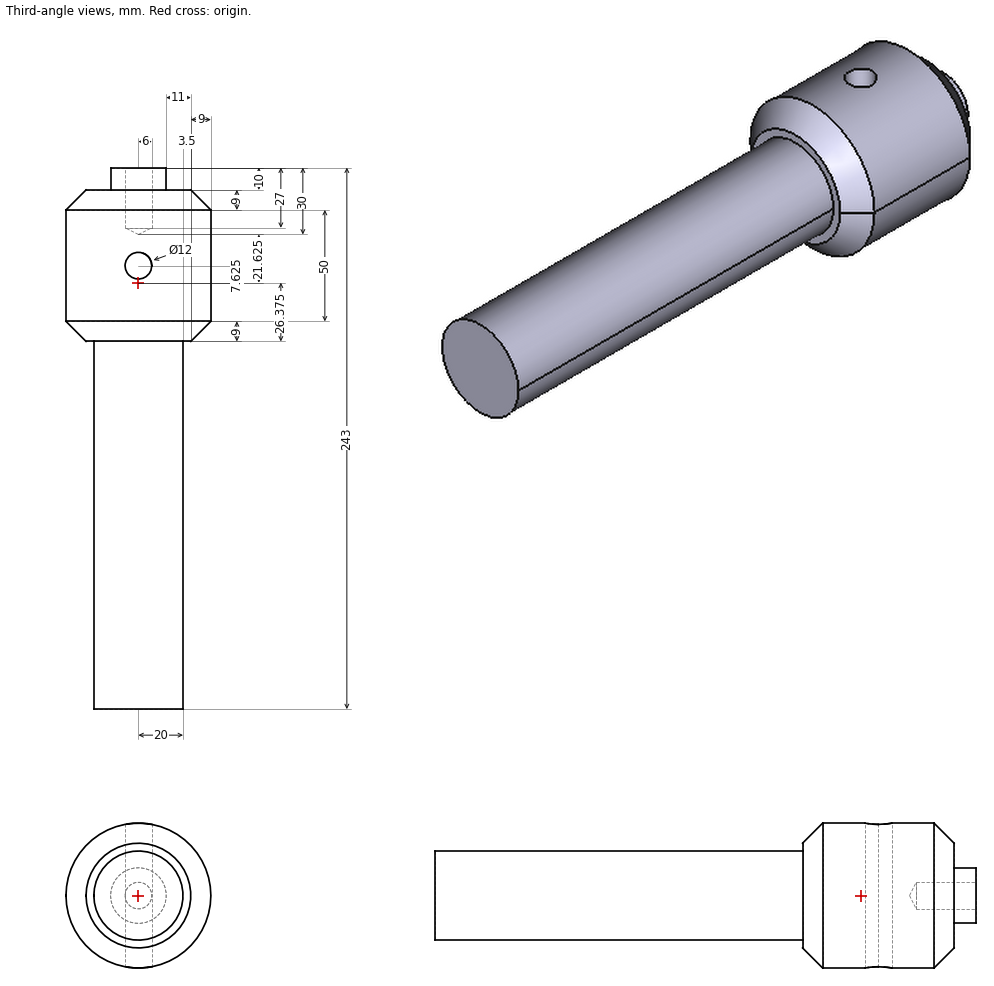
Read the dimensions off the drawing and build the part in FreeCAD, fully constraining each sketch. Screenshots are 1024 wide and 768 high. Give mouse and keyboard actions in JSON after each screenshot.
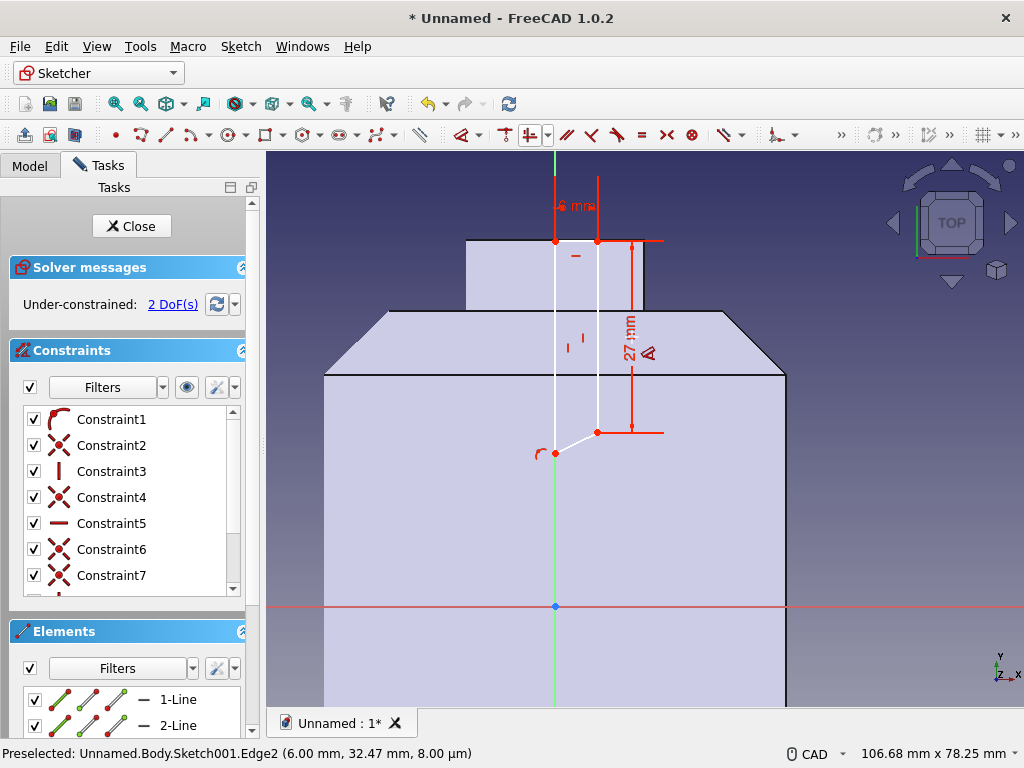
{"action": "left_click", "coordinate": [555, 305]}
{"action": "left_click", "coordinate": [521, 348]}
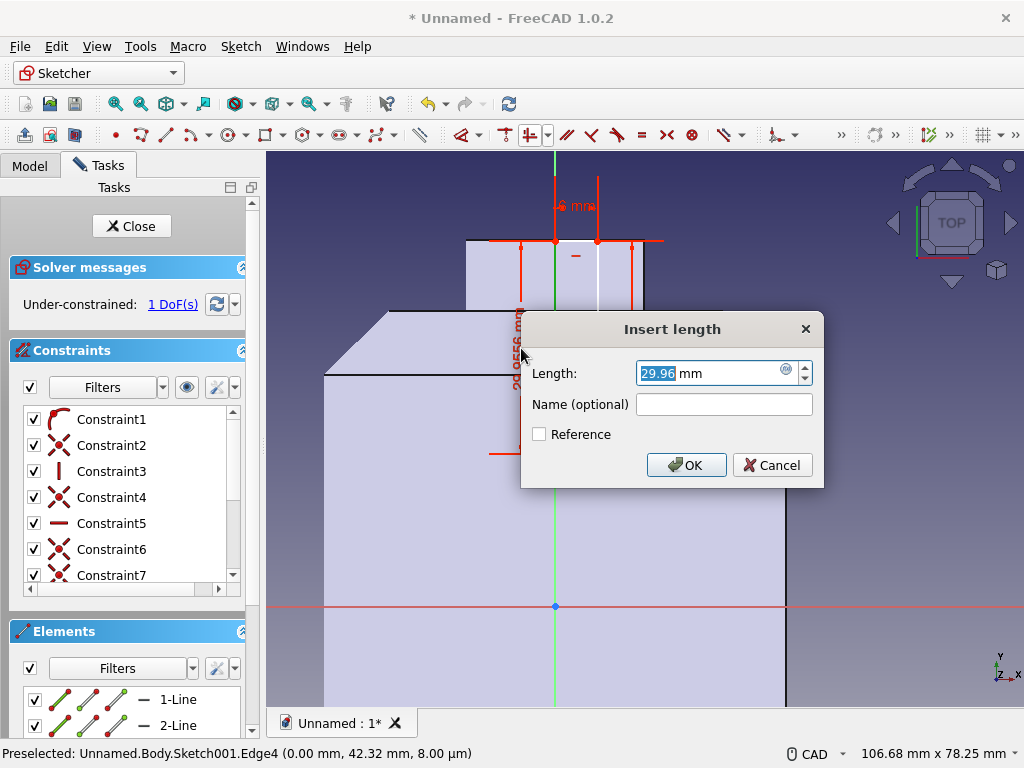
{"action": "type", "text": "30"}
{"action": "key", "text": "Return"}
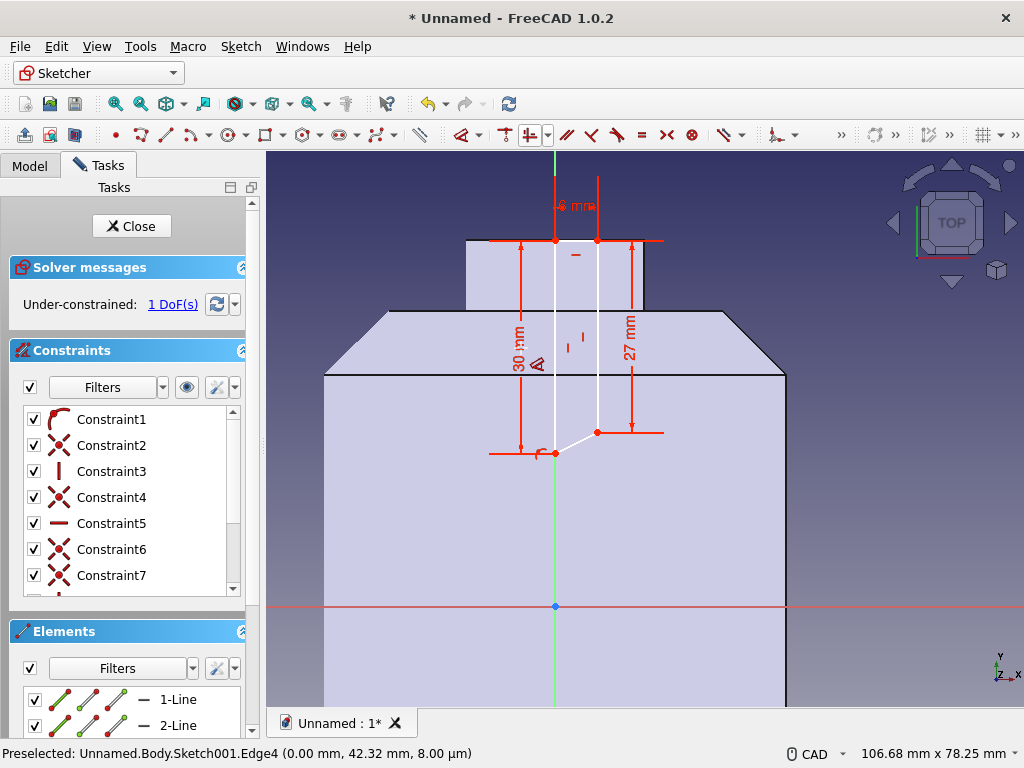
{"action": "left_click", "coordinate": [555, 454]}
{"action": "left_click", "coordinate": [521, 530]}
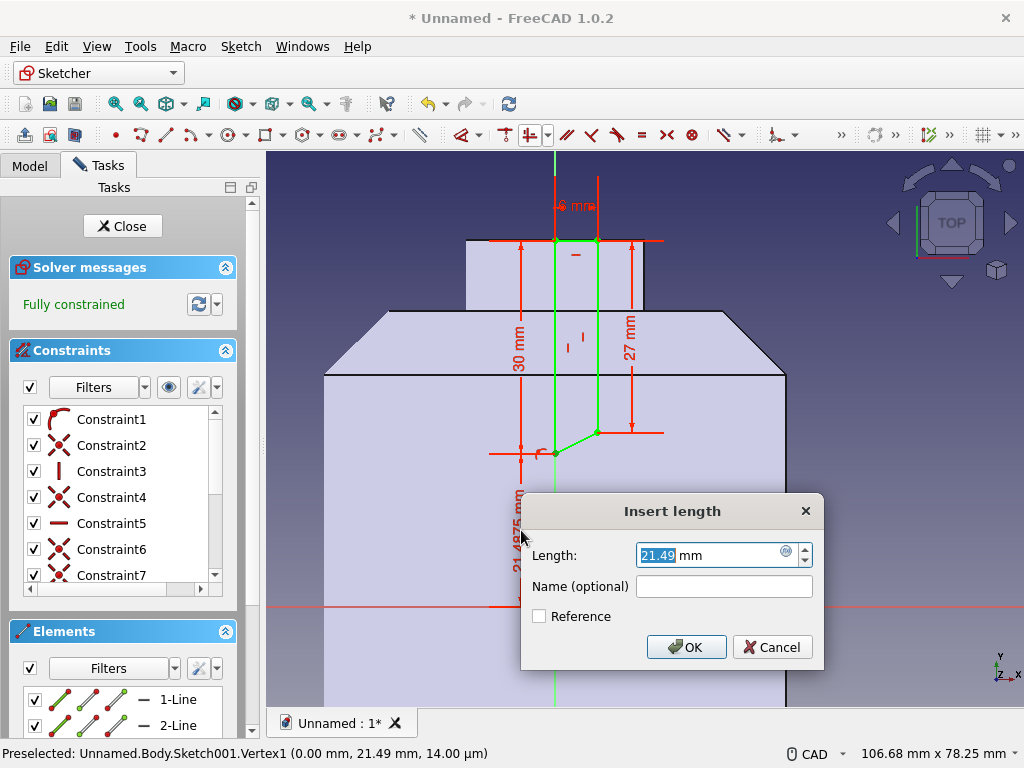
{"action": "type", "text": "21.625"}
{"action": "key", "text": "Return"}
{"action": "key", "text": "Escape"}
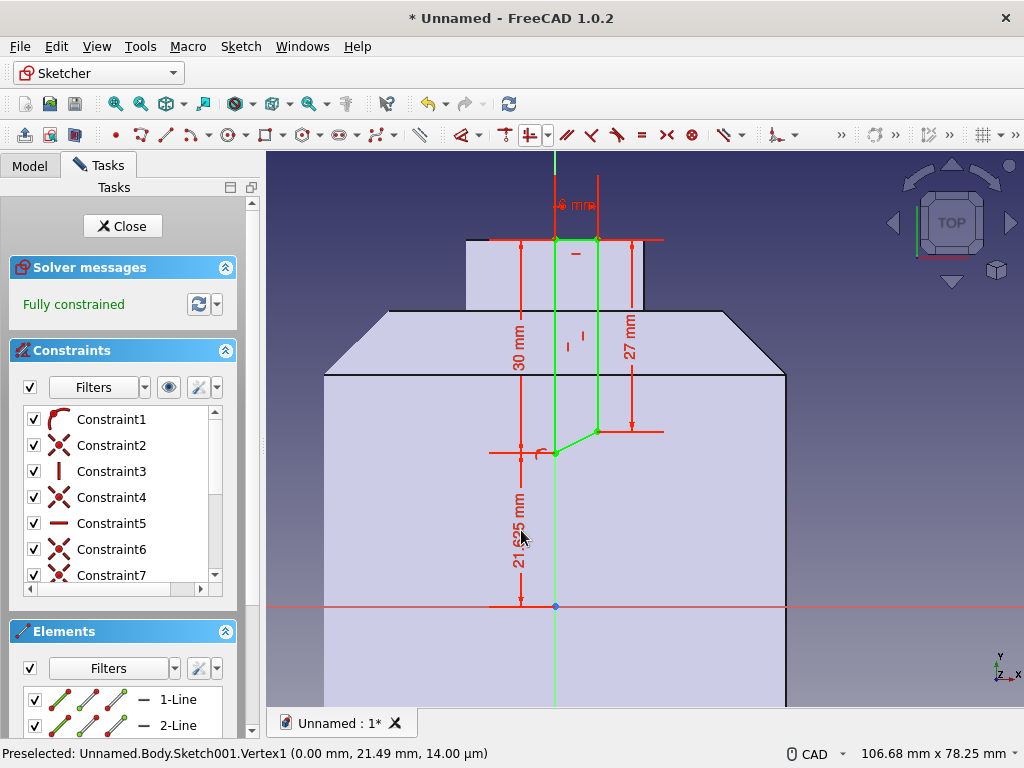
{"action": "left_click", "coordinate": [123, 226]}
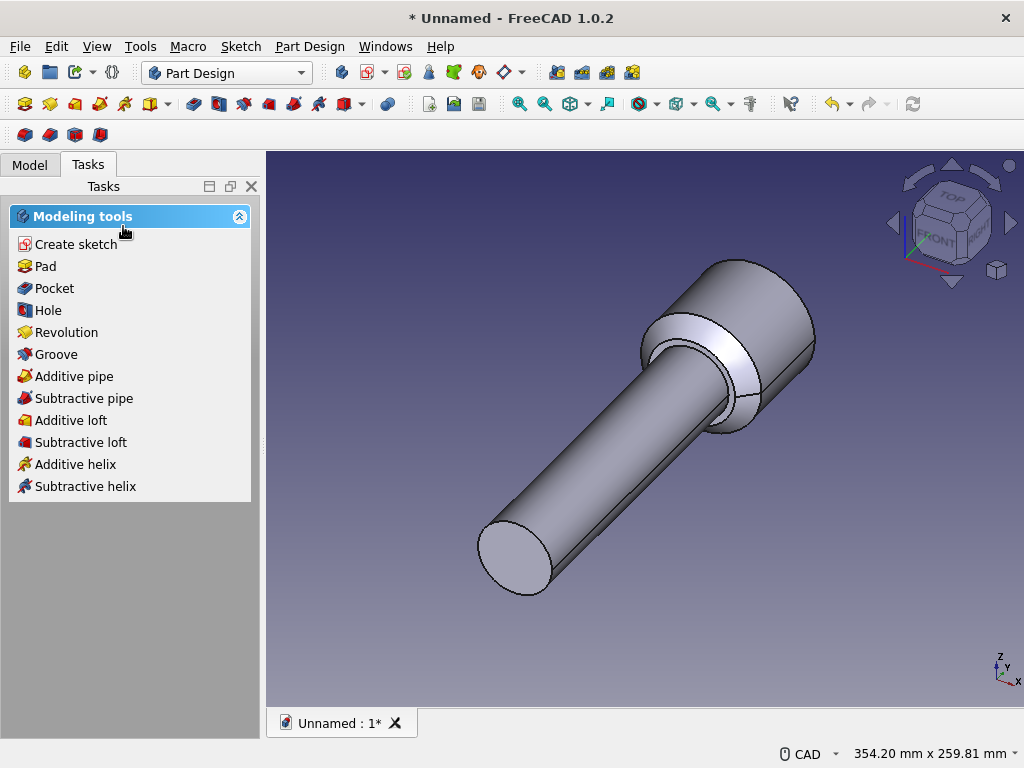
{"action": "left_click", "coordinate": [244, 104]}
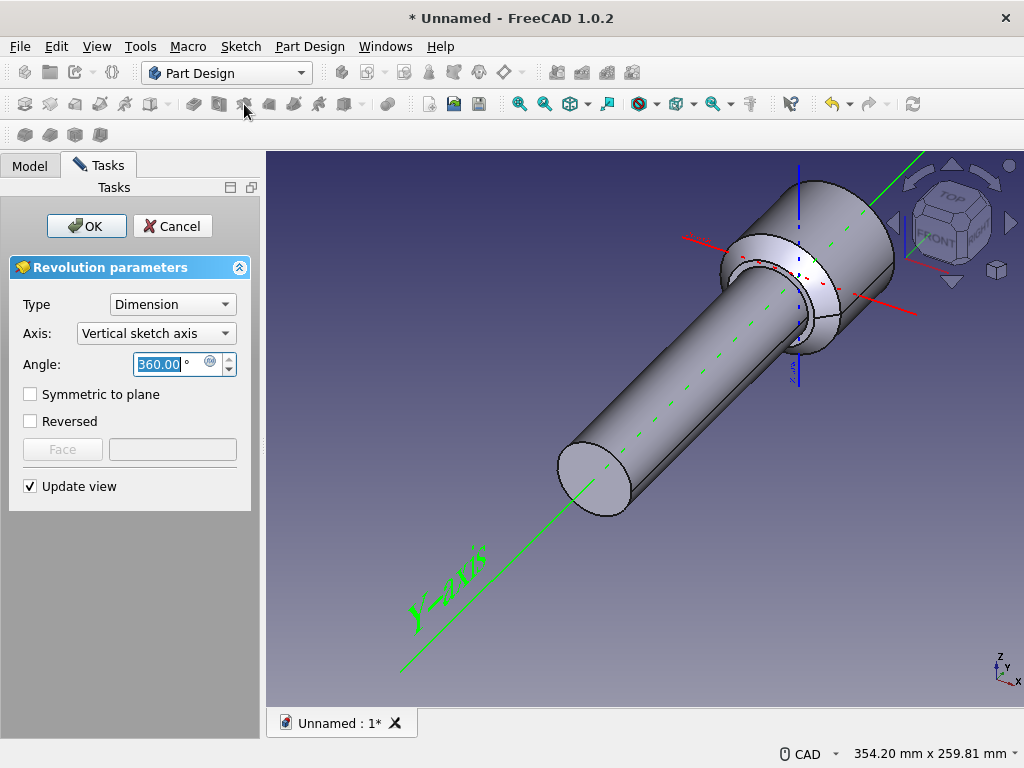
{"action": "left_click", "coordinate": [87, 226]}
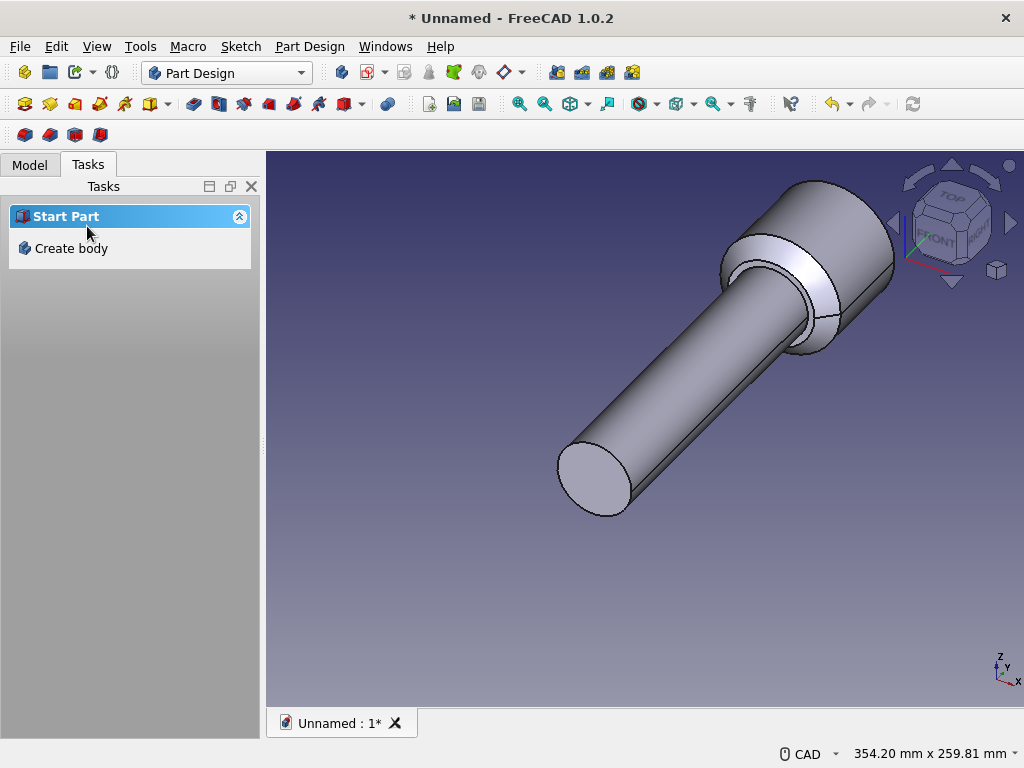
{"action": "left_click", "coordinate": [520, 104]}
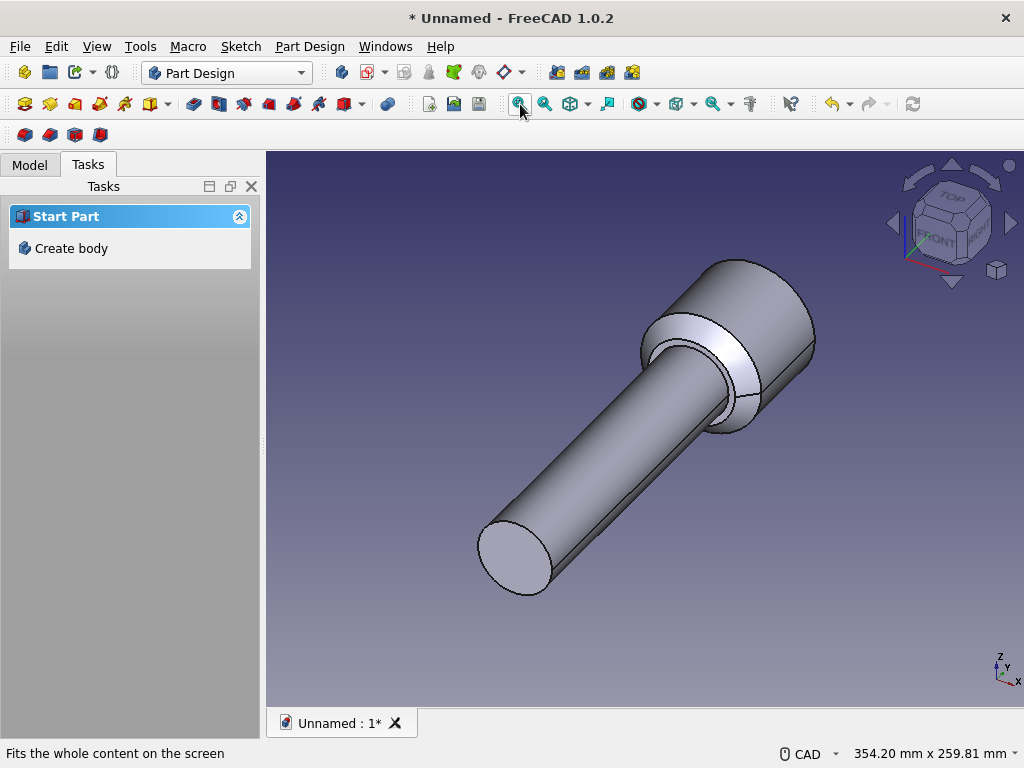
{"action": "left_click", "coordinate": [366, 72]}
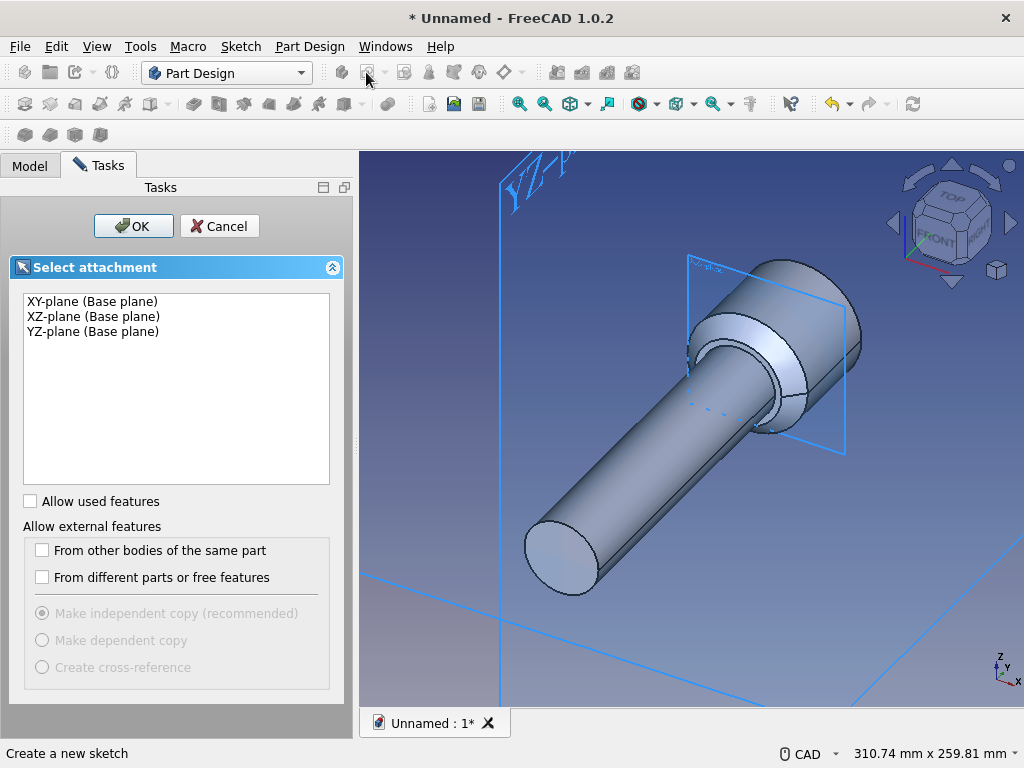
{"action": "left_click", "coordinate": [84, 302]}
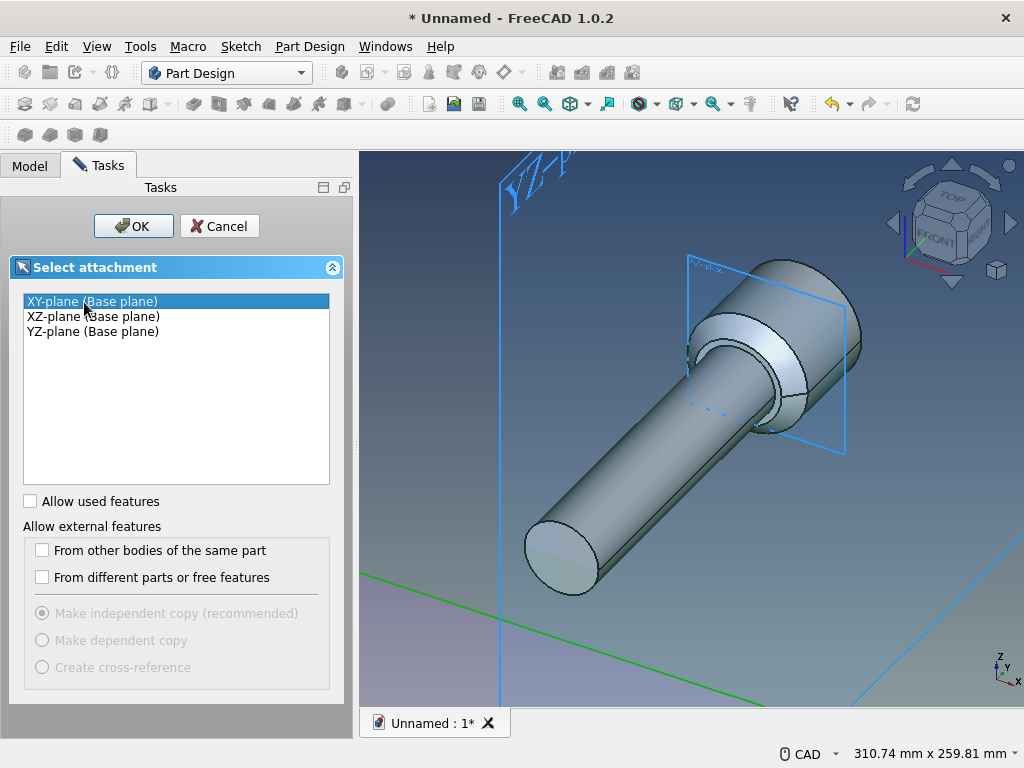
{"action": "left_click", "coordinate": [134, 226]}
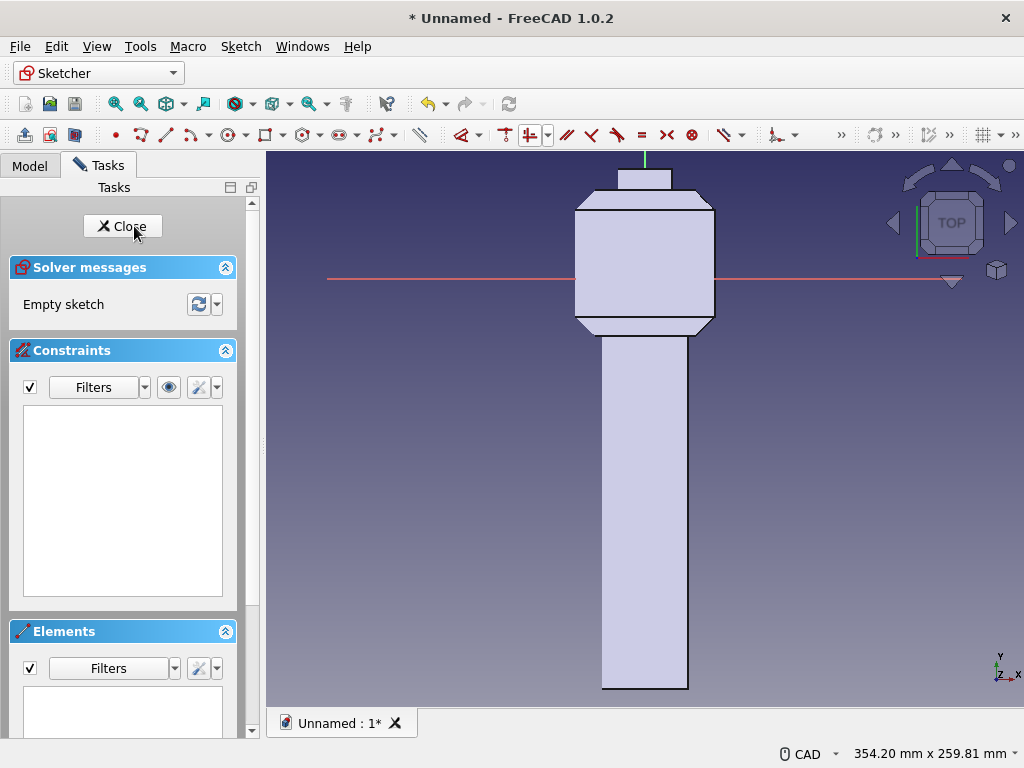
{"action": "left_click", "coordinate": [75, 136]}